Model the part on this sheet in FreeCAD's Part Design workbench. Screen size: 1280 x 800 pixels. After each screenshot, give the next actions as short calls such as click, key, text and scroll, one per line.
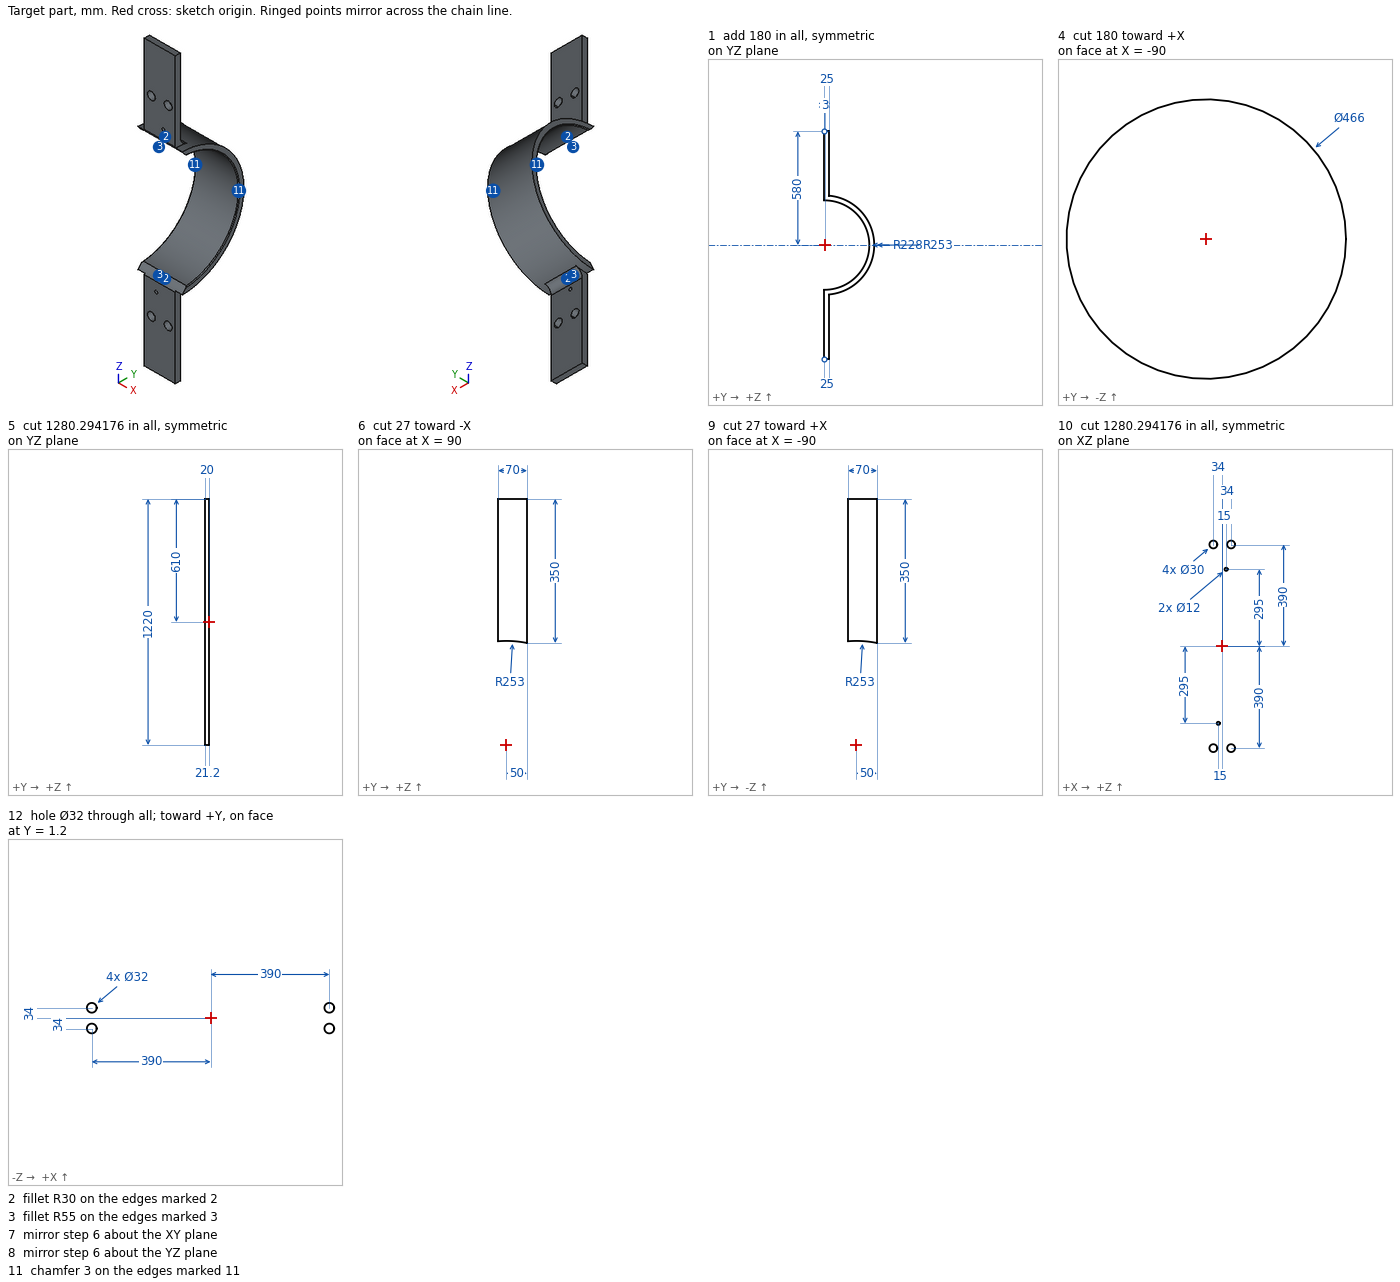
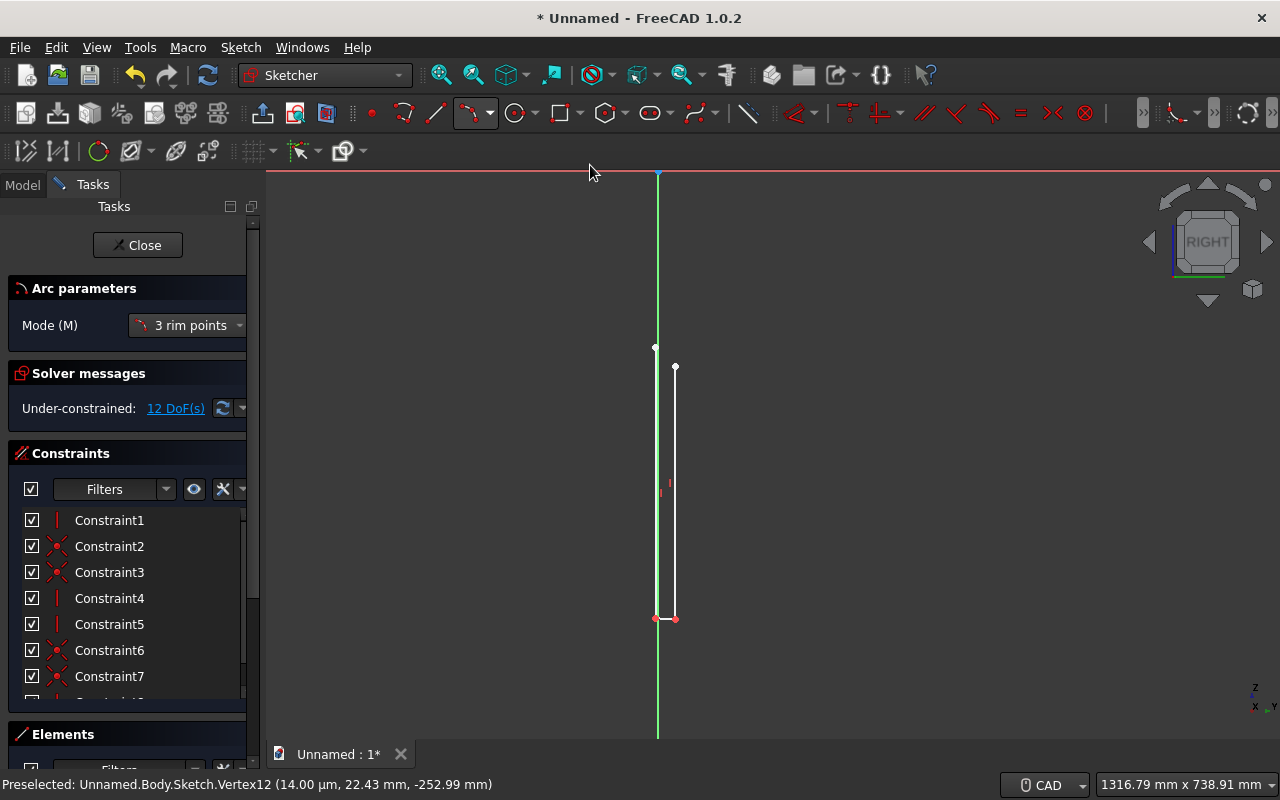
scroll(676, 619, down, 5)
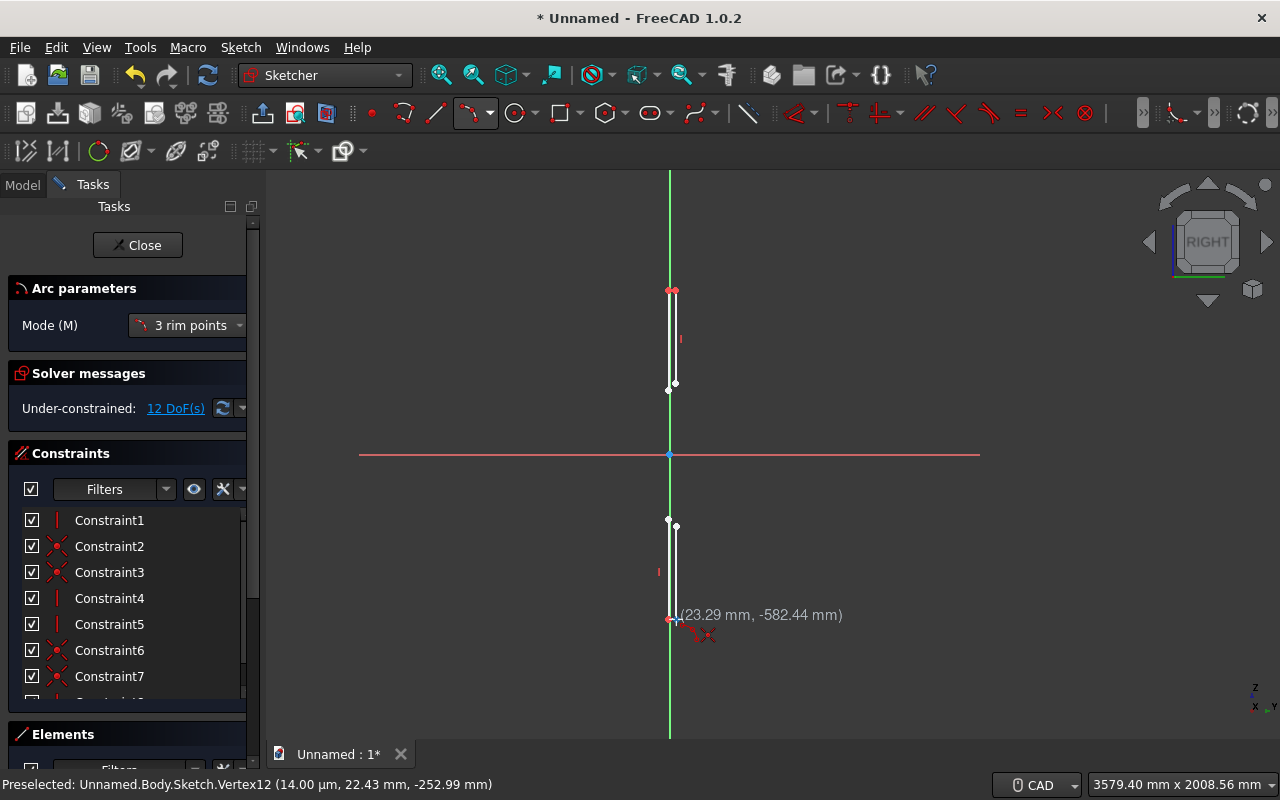
scroll(669, 390, up, 15)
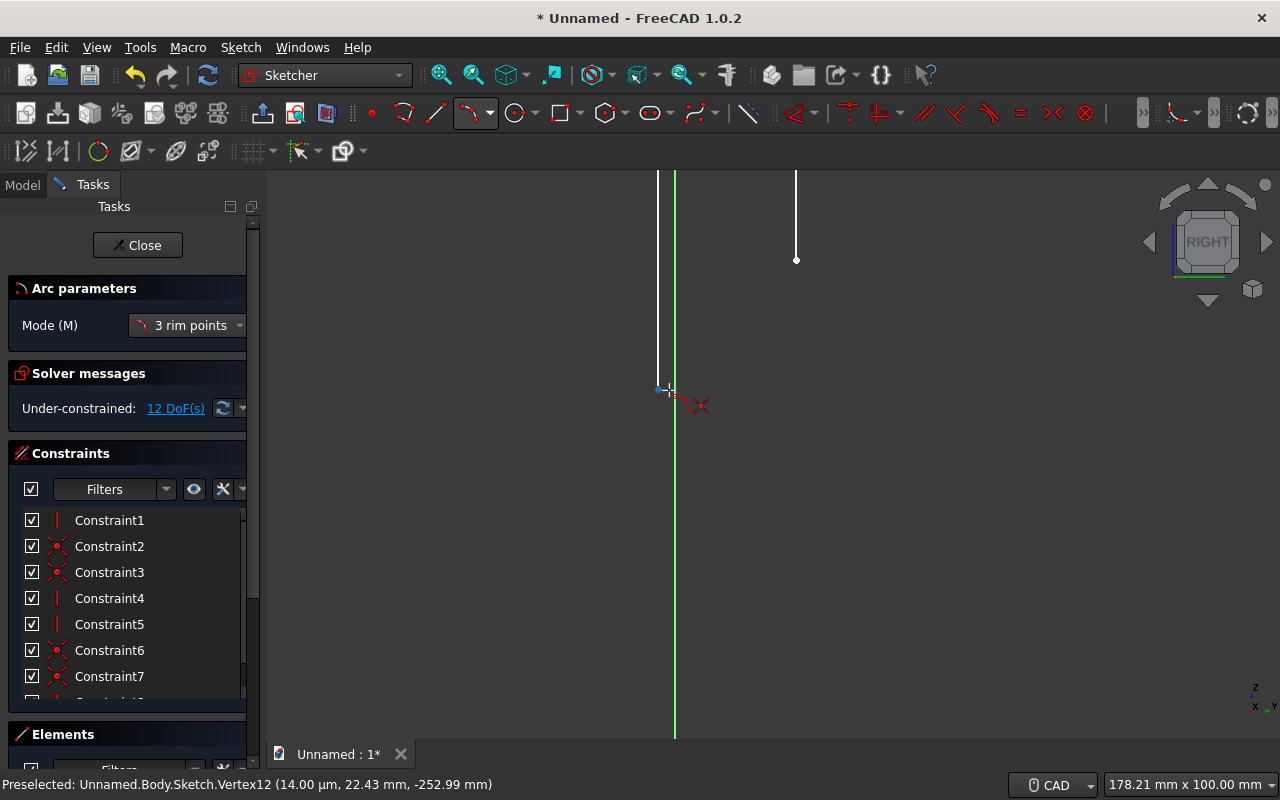
click(658, 389)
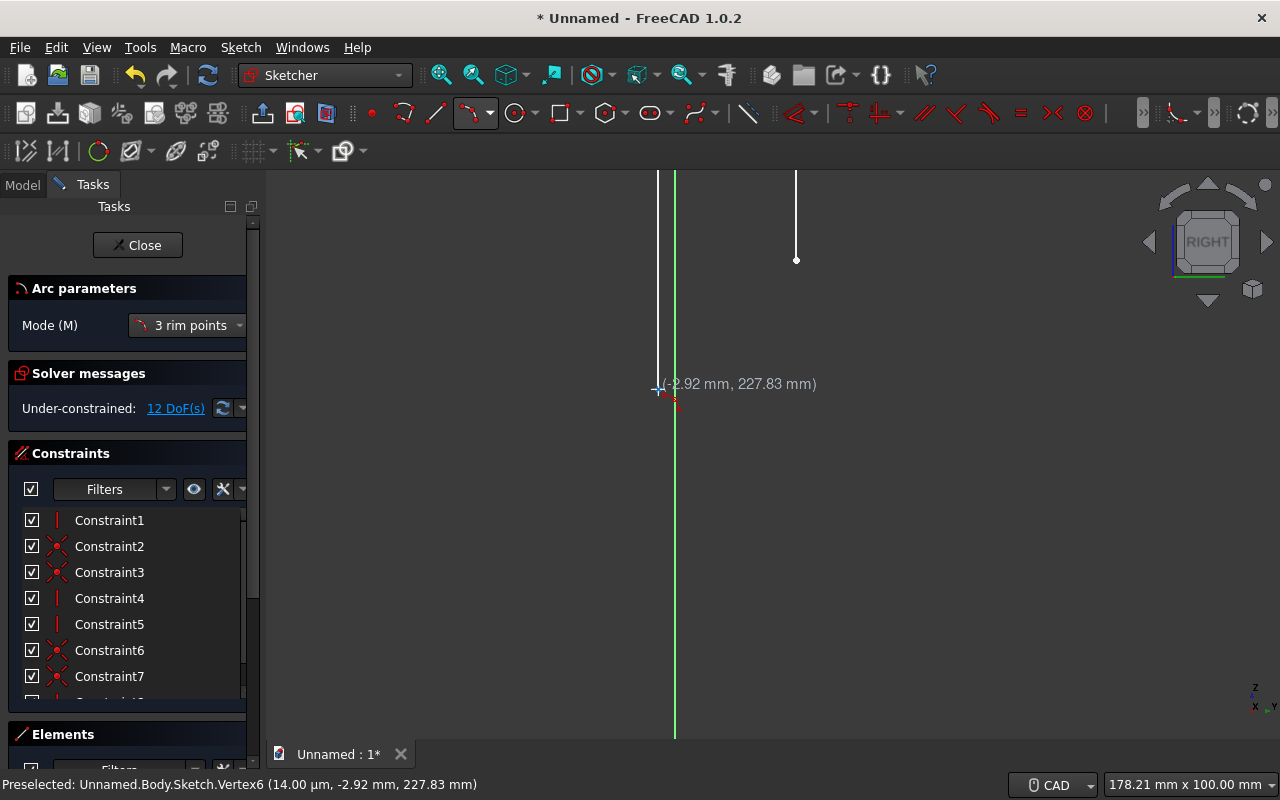
scroll(669, 390, down, 15)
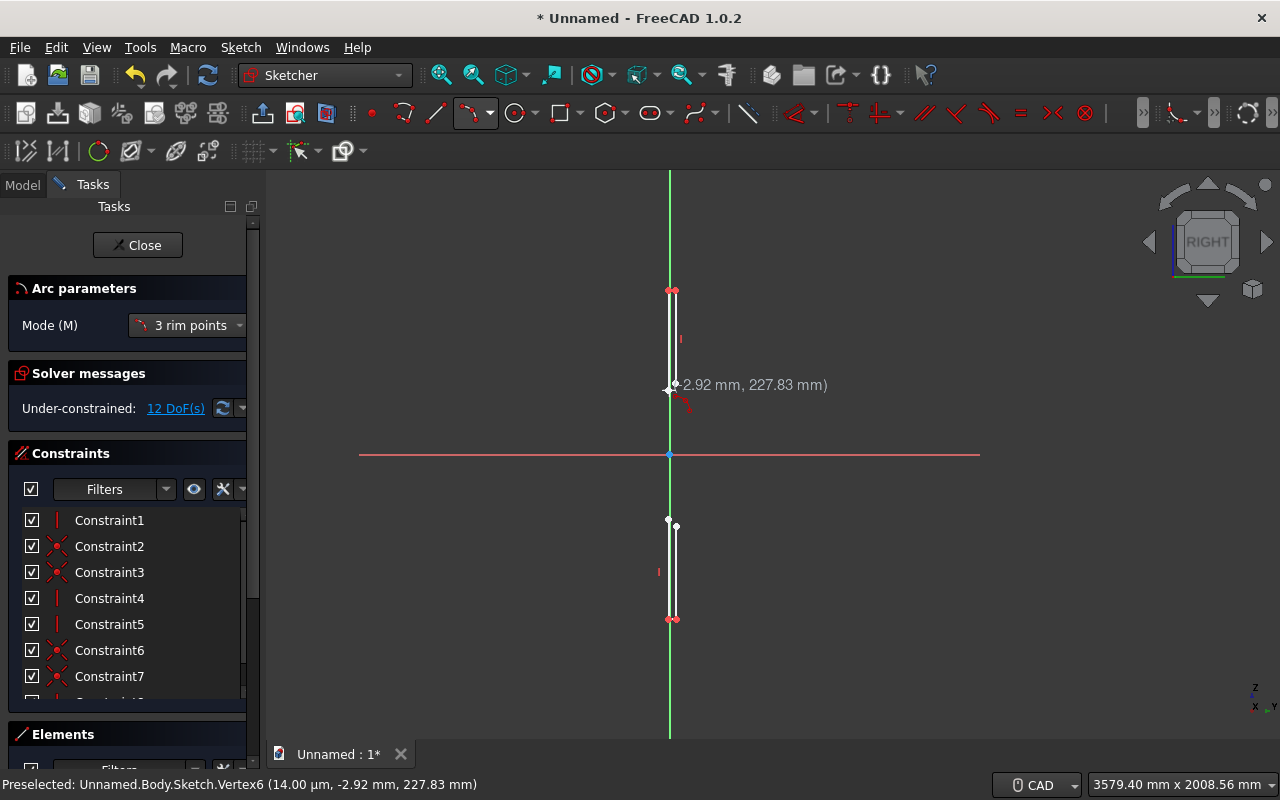
scroll(669, 519, up, 15)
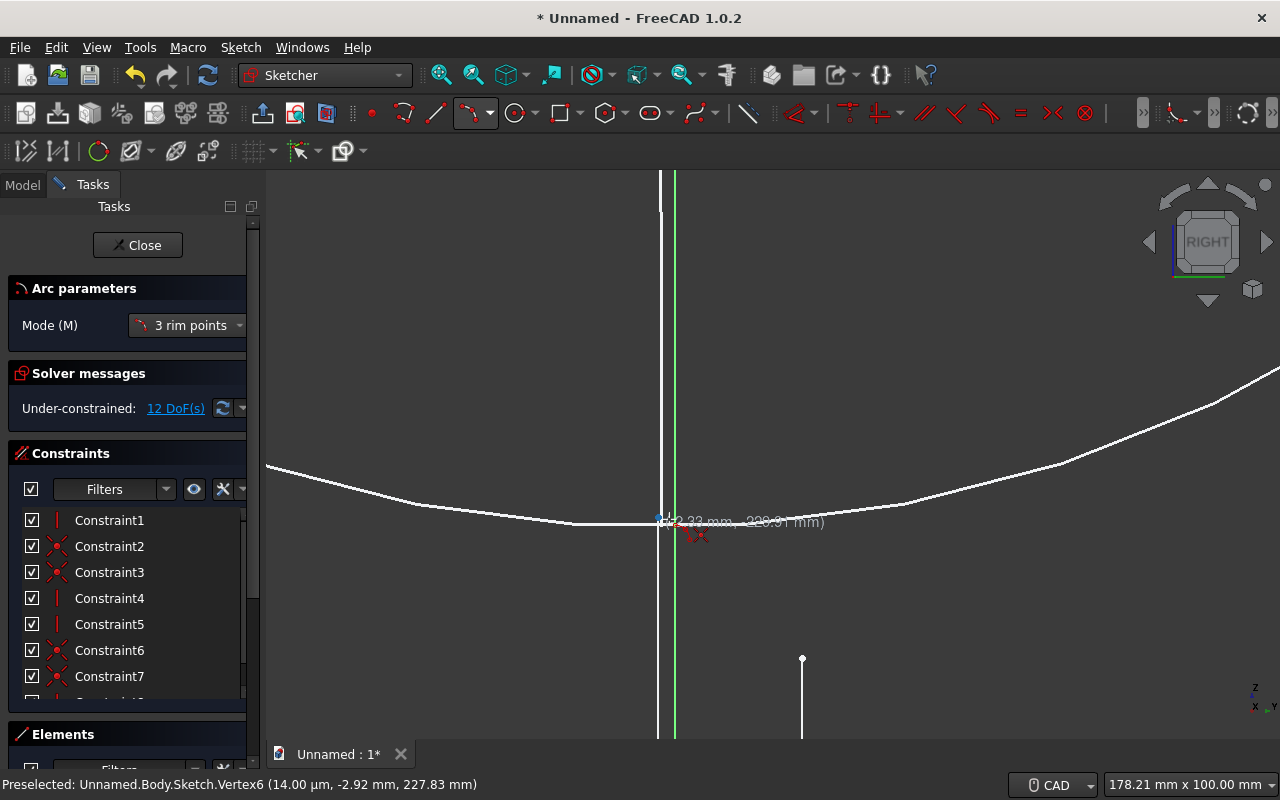
click(658, 517)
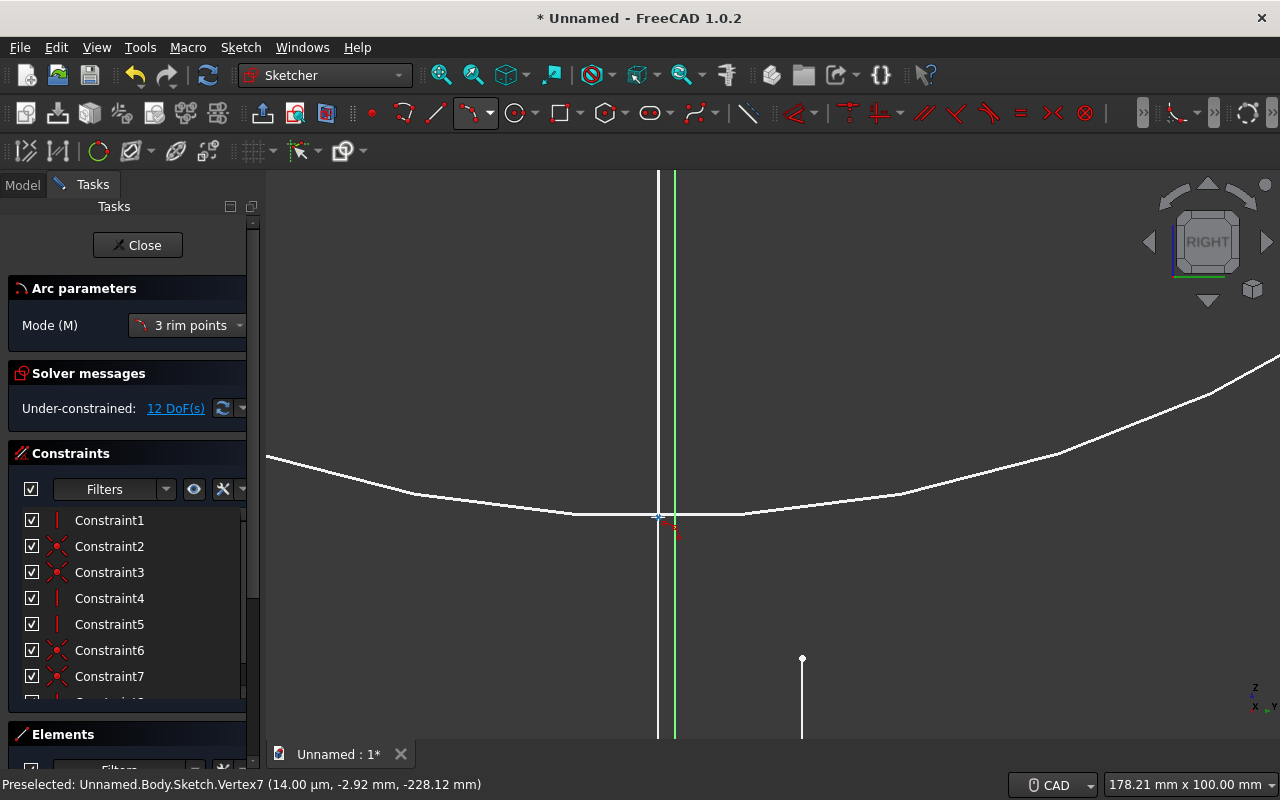
scroll(669, 519, down, 15)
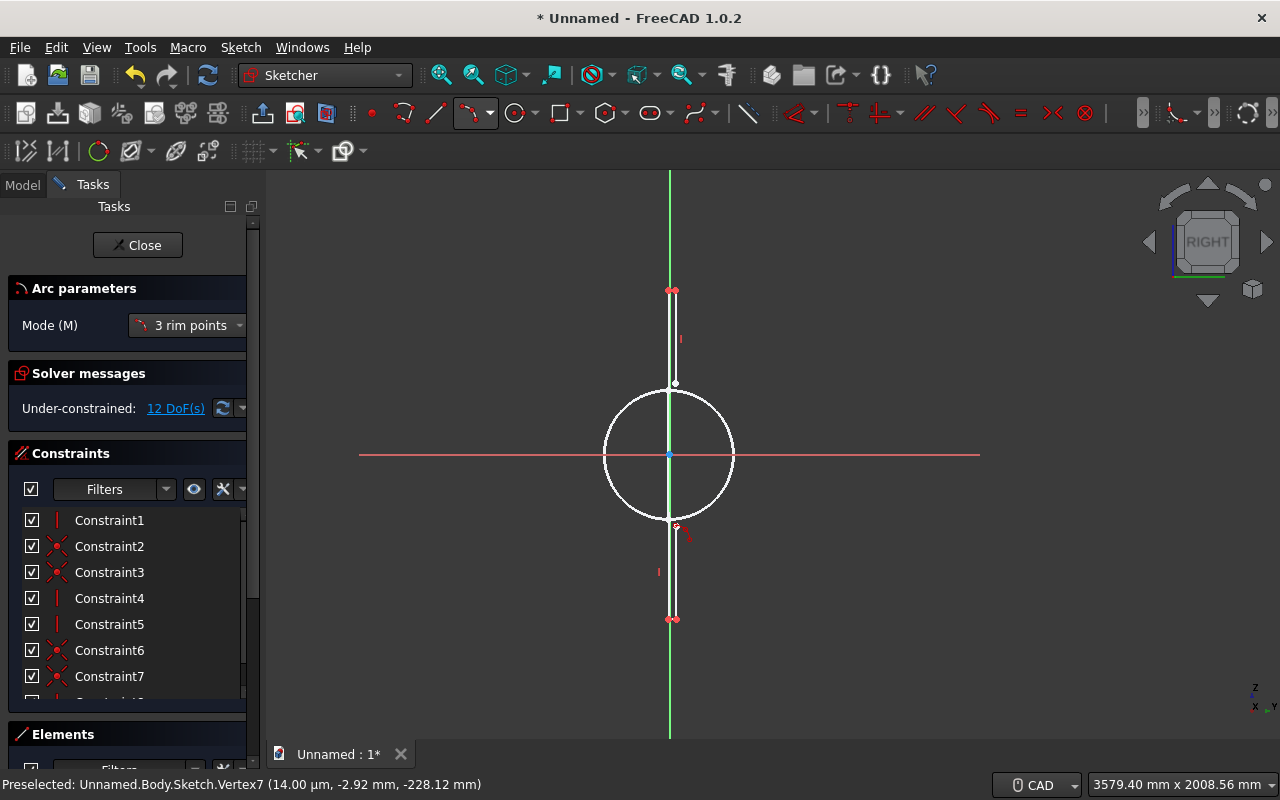
click(731, 475)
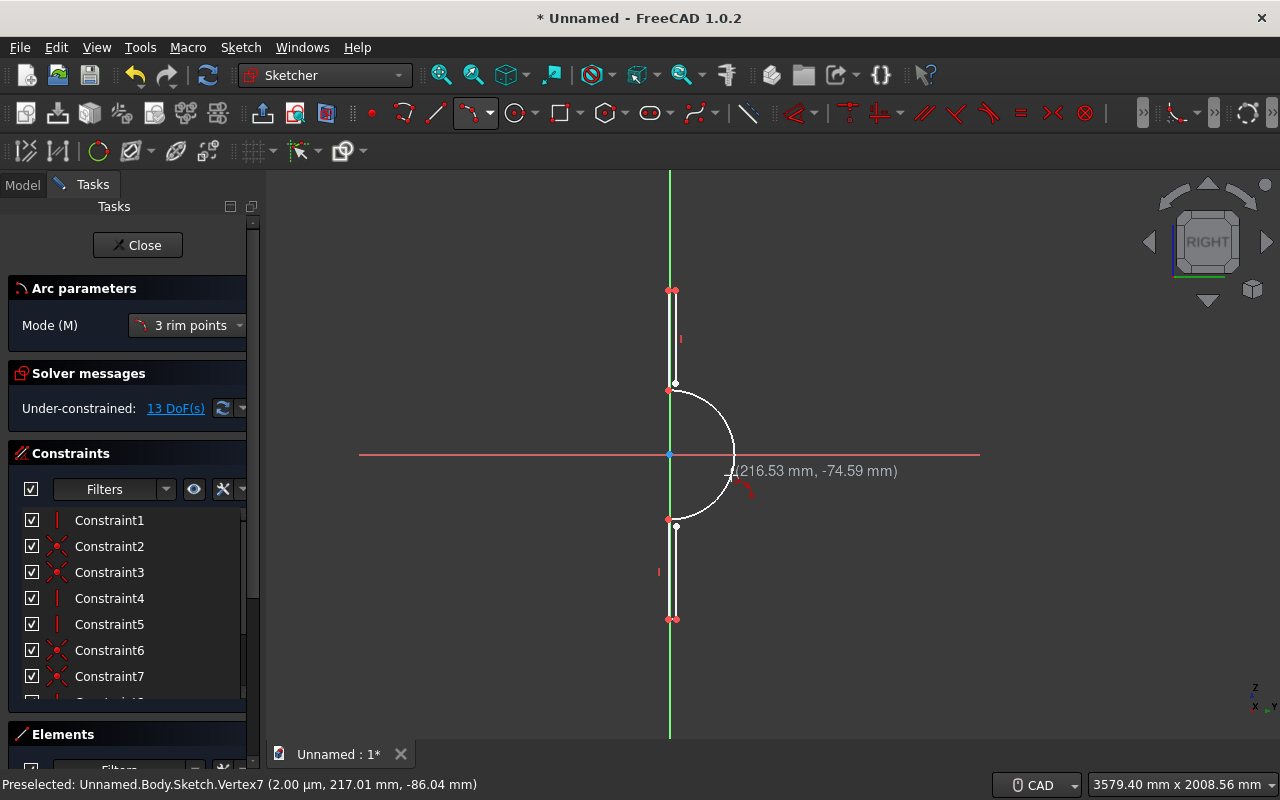
scroll(676, 526, up, 5)